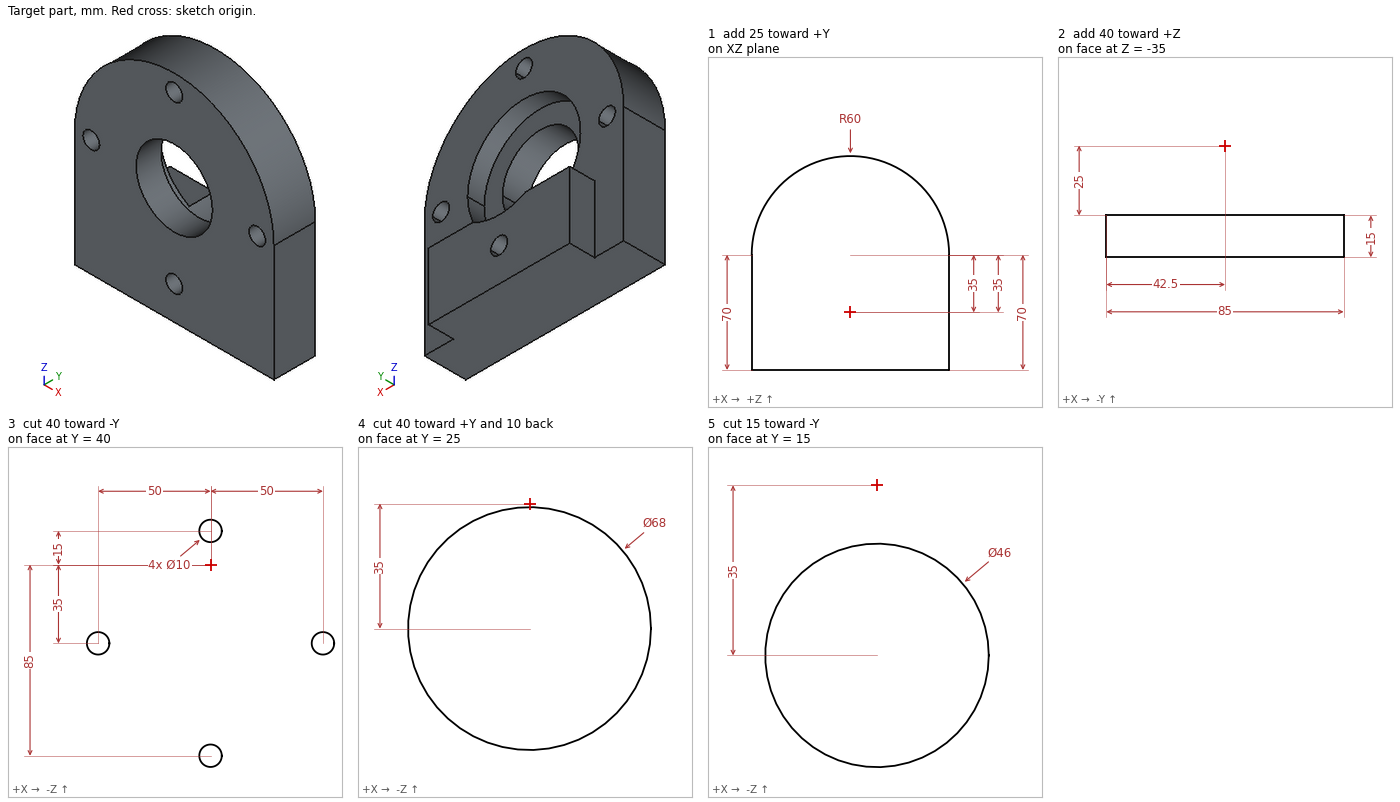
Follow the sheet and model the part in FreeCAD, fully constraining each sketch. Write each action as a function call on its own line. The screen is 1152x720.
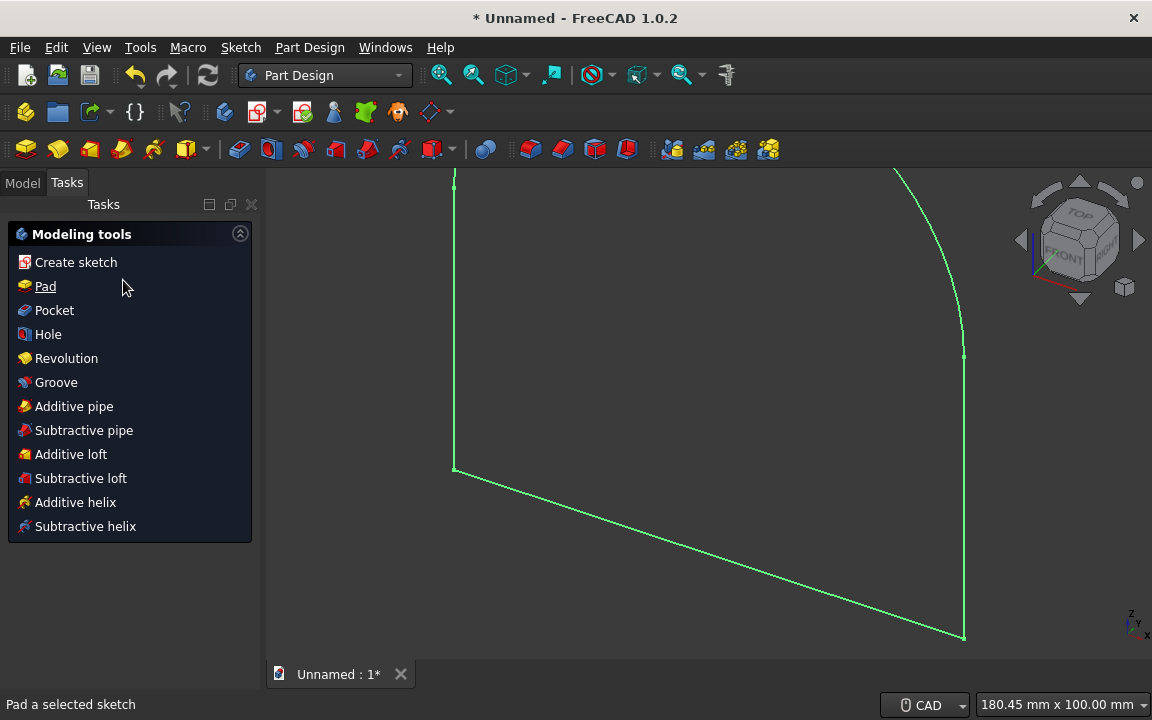
click(26, 150)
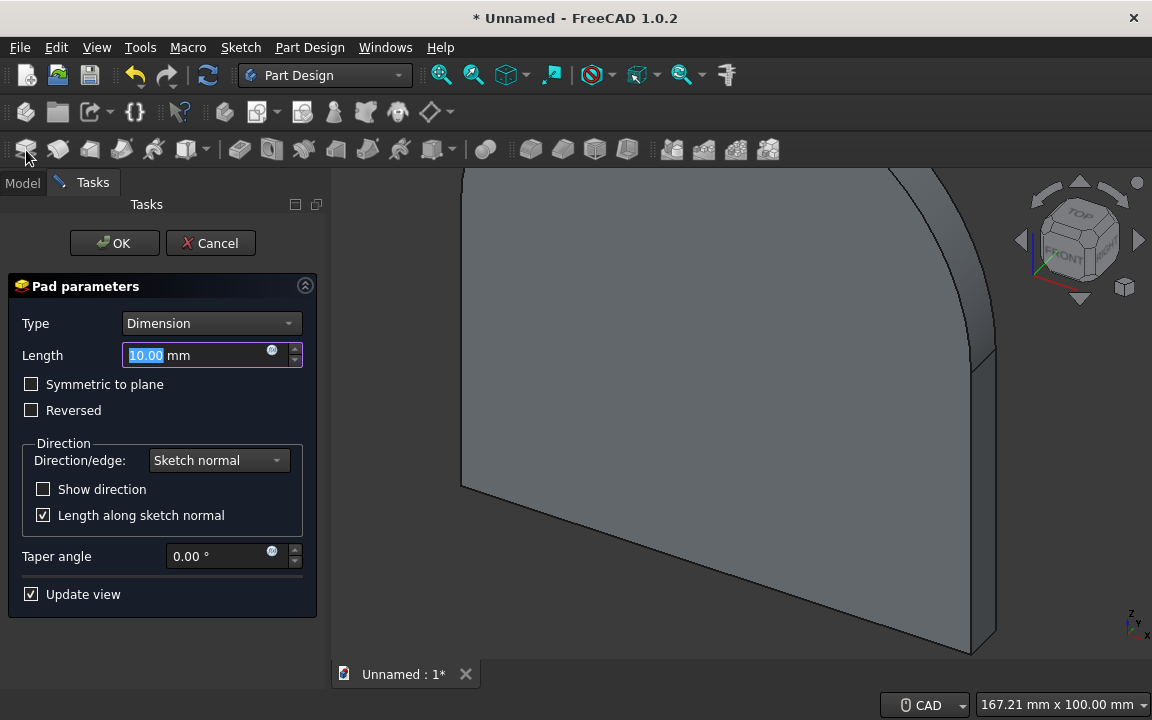
text(25)
key(Tab)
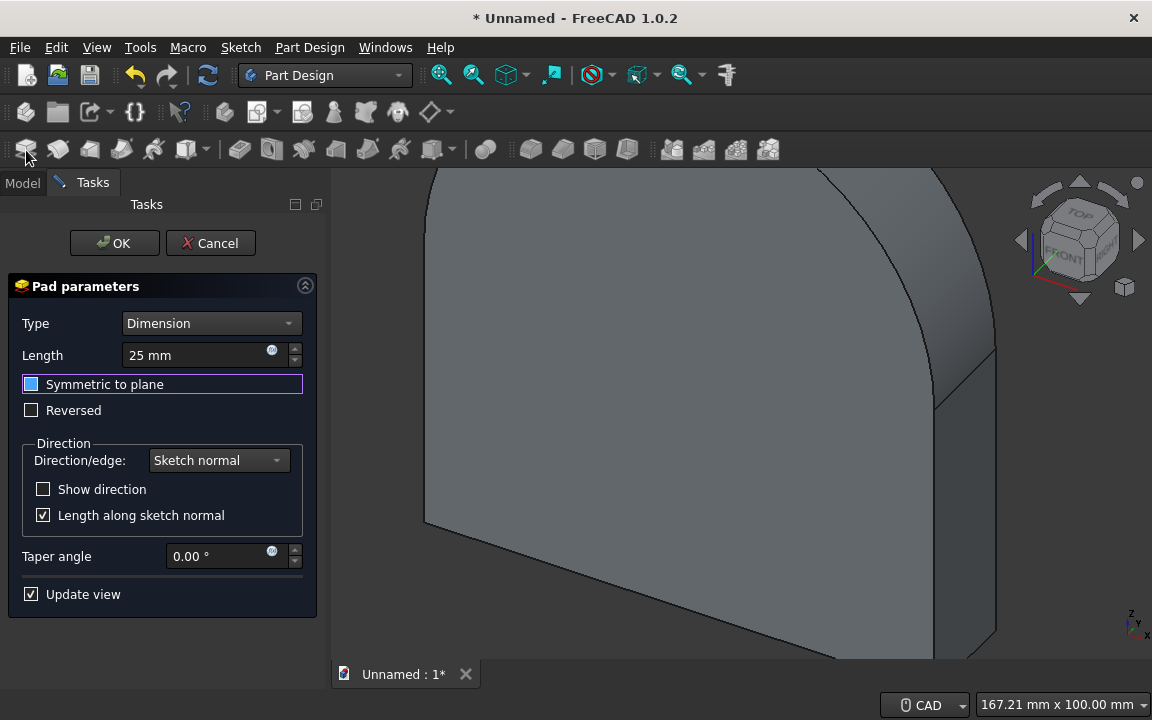
click(30, 410)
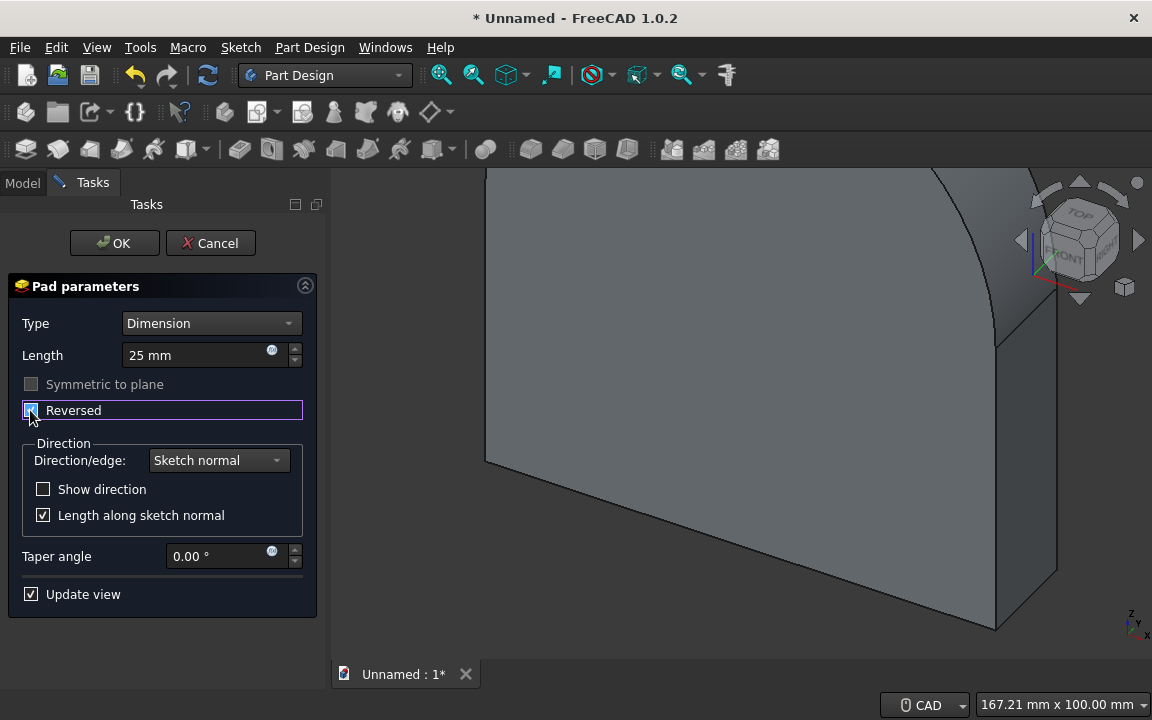
click(115, 243)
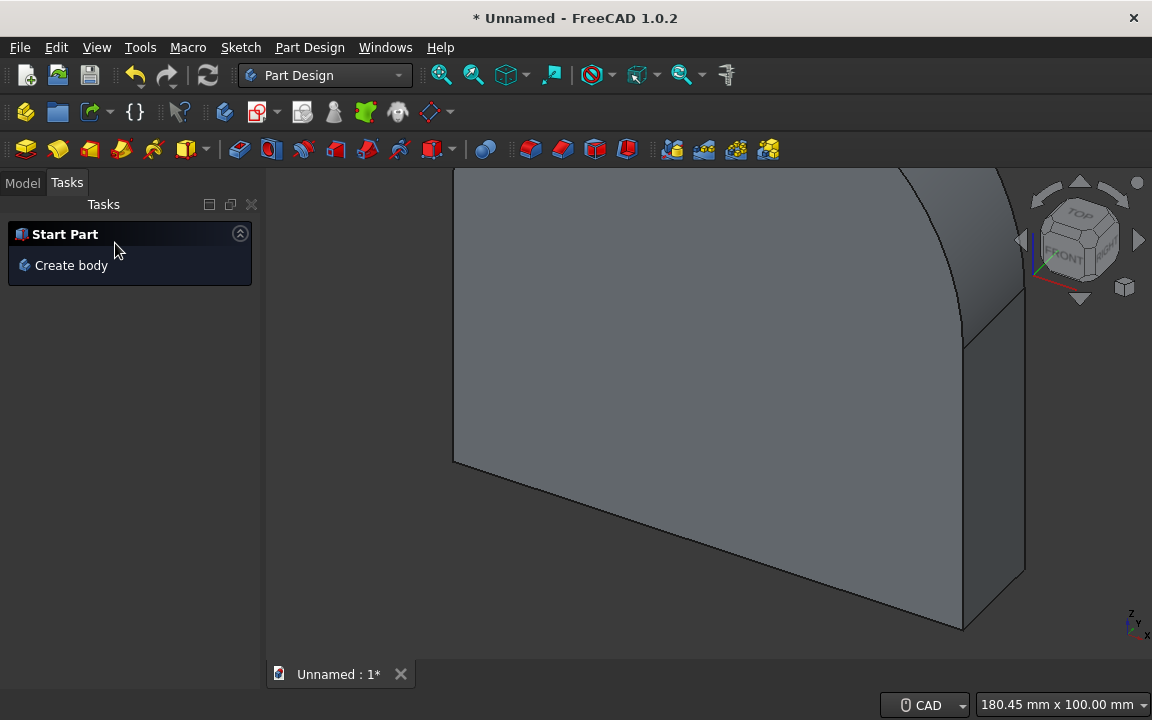
click(442, 76)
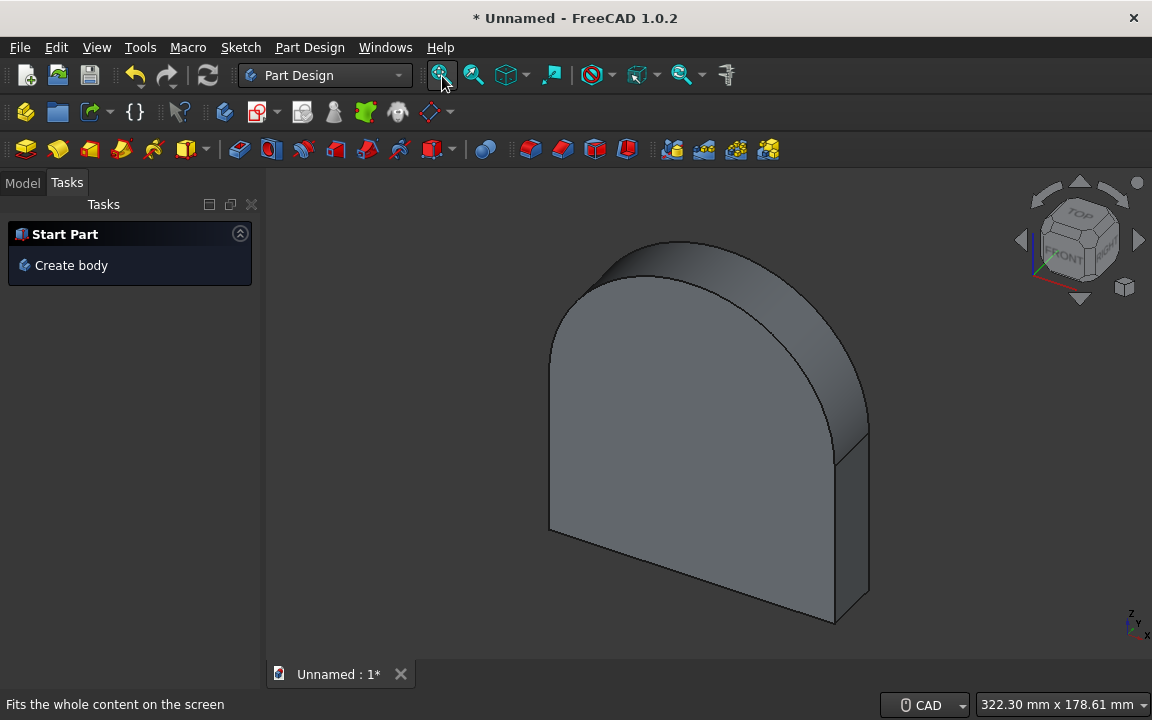
key(5)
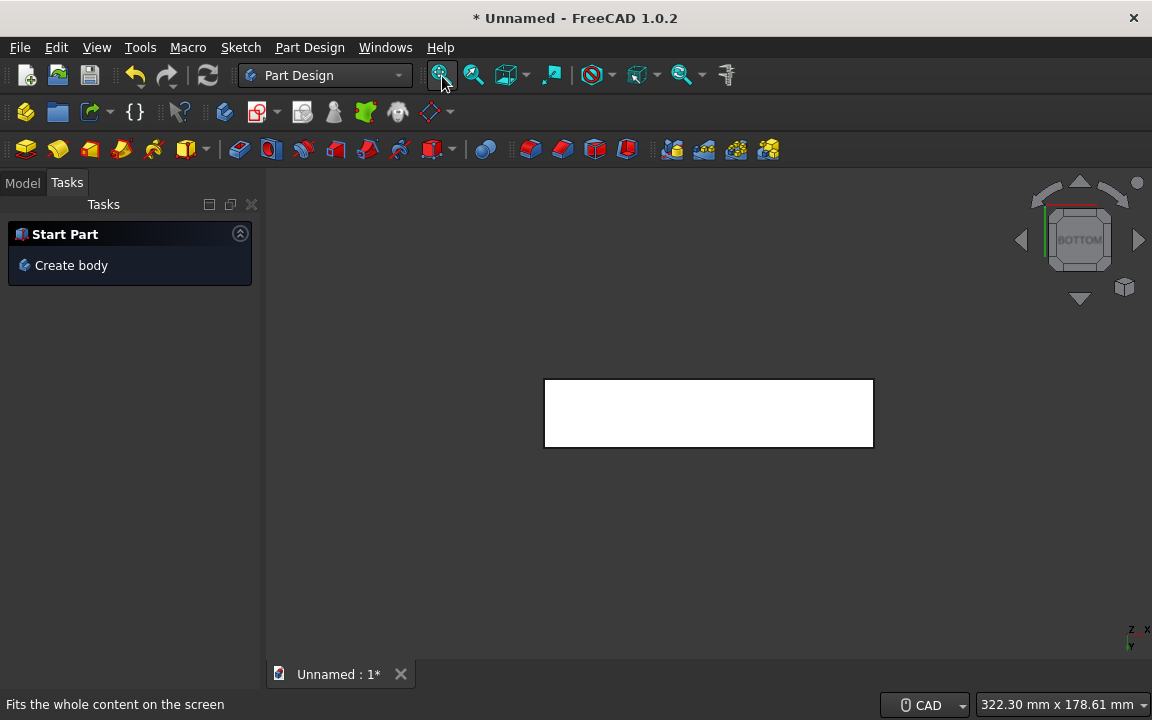
click(442, 76)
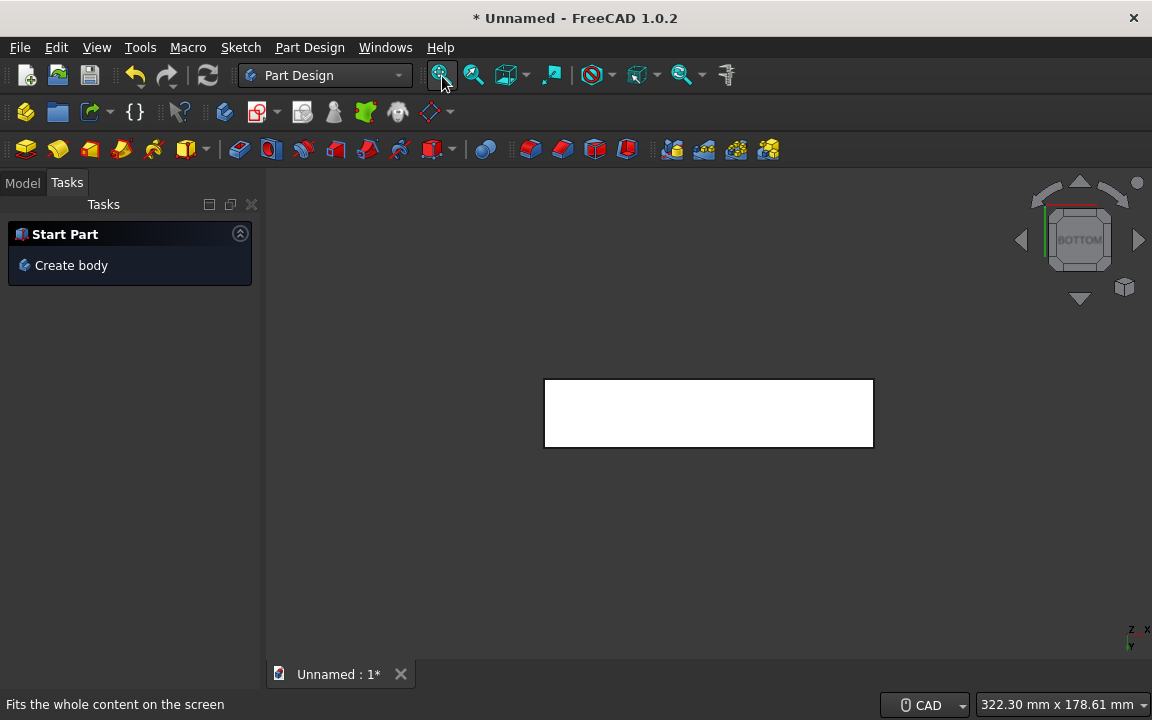
click(803, 412)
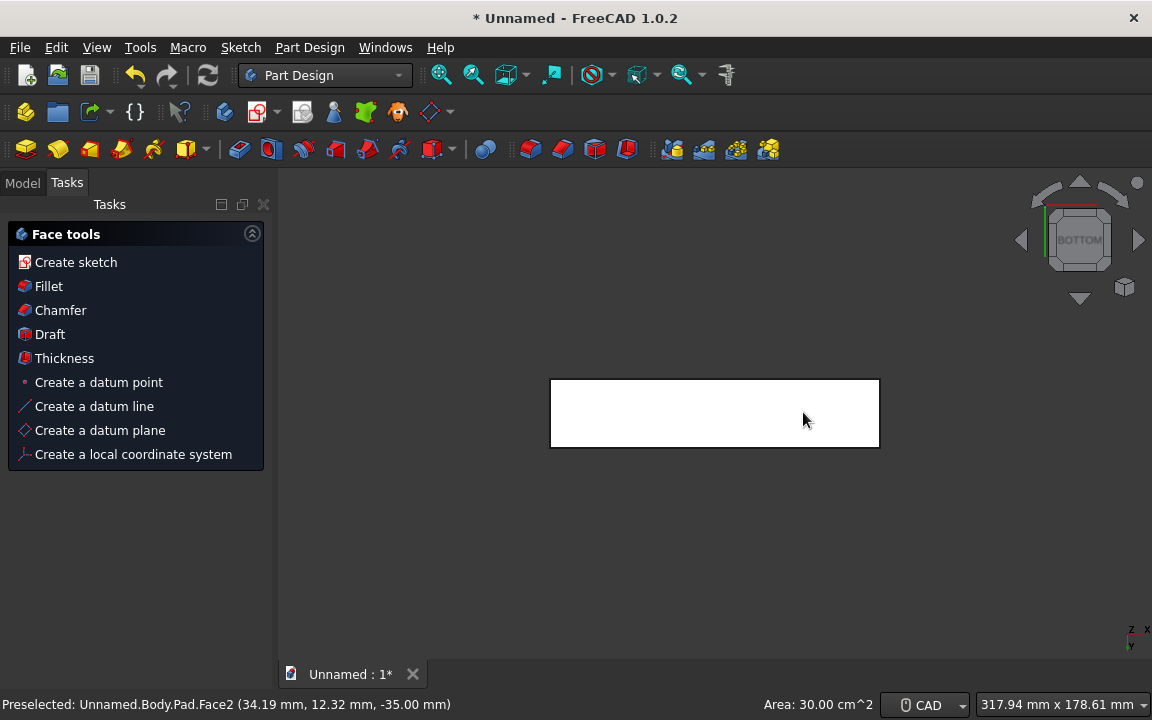
click(258, 112)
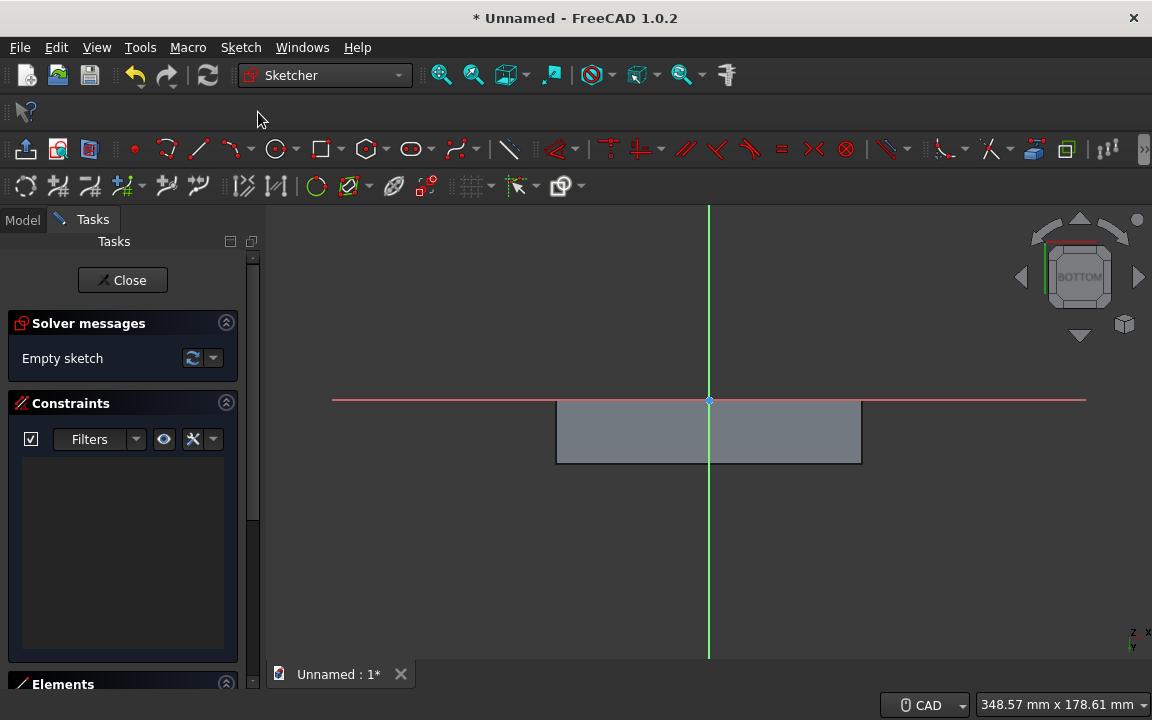
scroll(765, 467, up, 4)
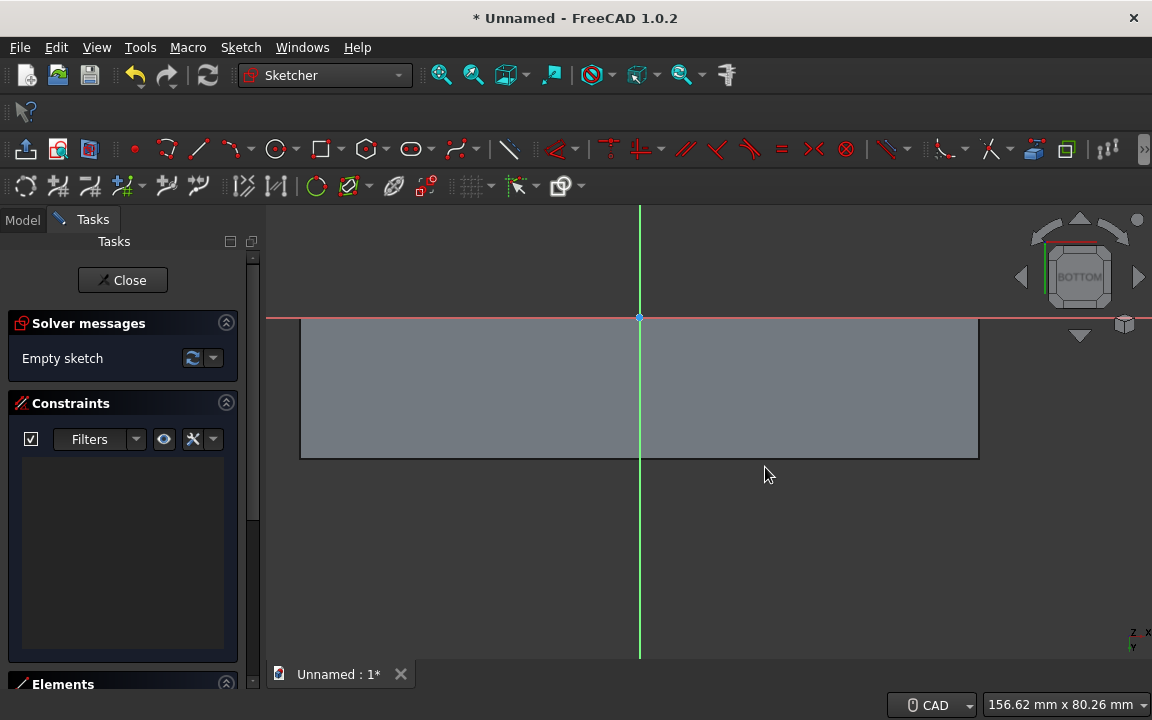
key(g)
key(r)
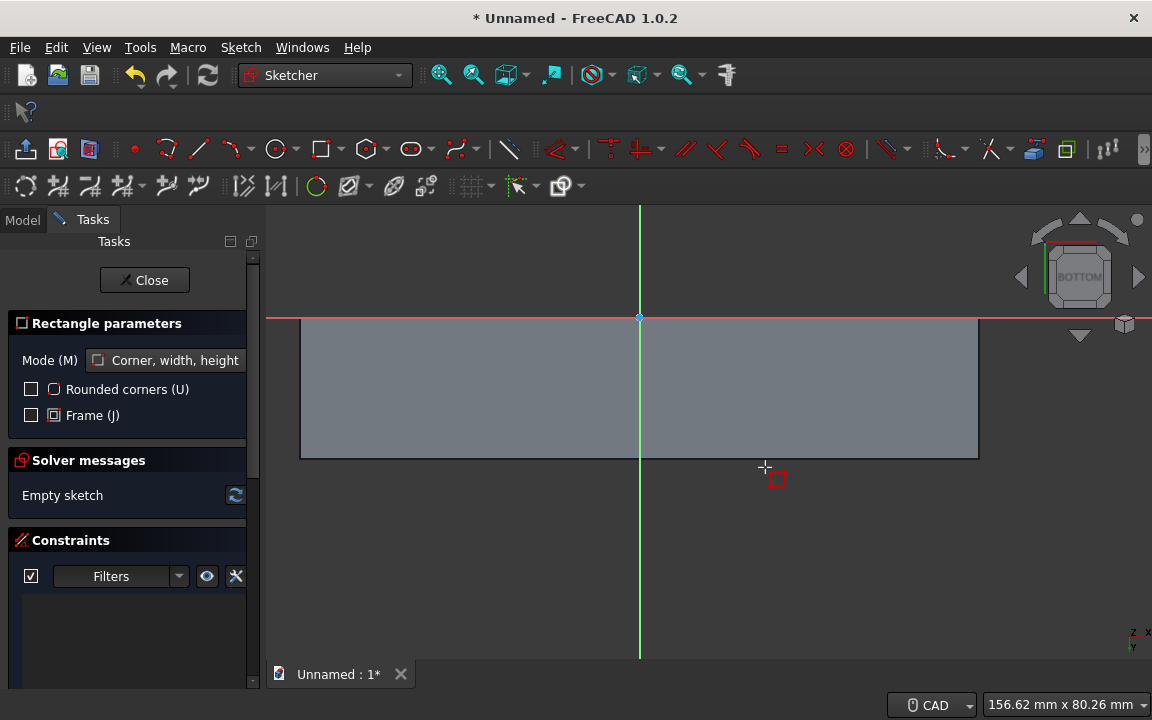
click(399, 459)
move(880, 544)